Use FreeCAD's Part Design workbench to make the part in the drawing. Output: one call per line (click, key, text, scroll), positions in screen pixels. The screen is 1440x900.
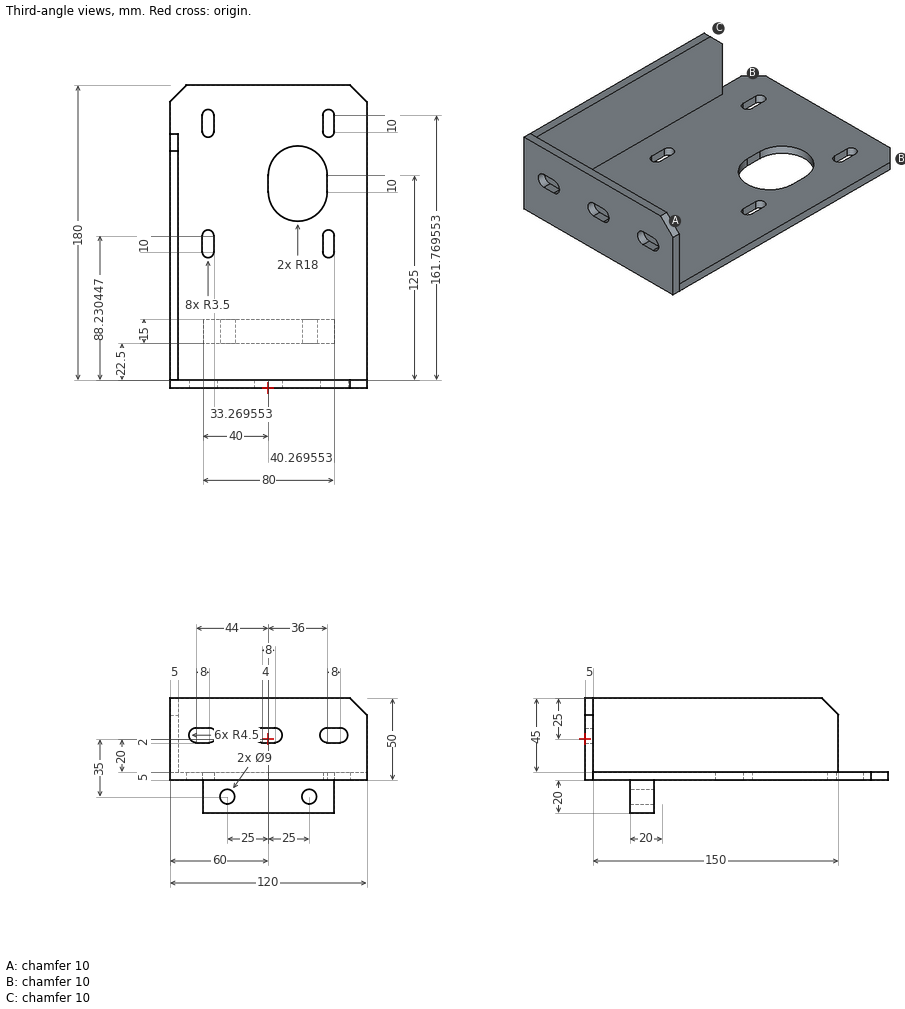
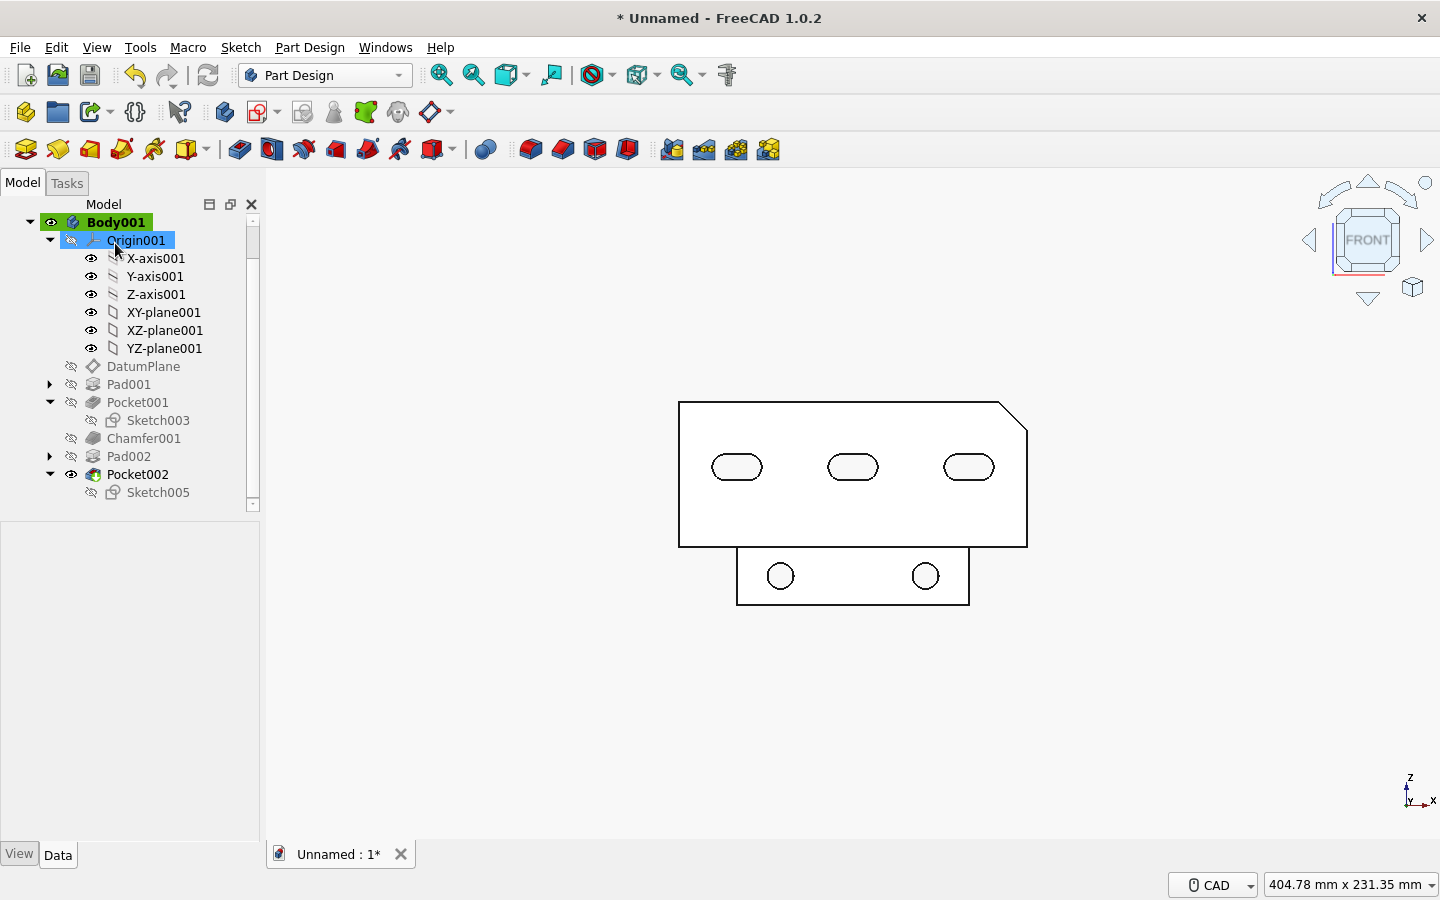
click(226, 112)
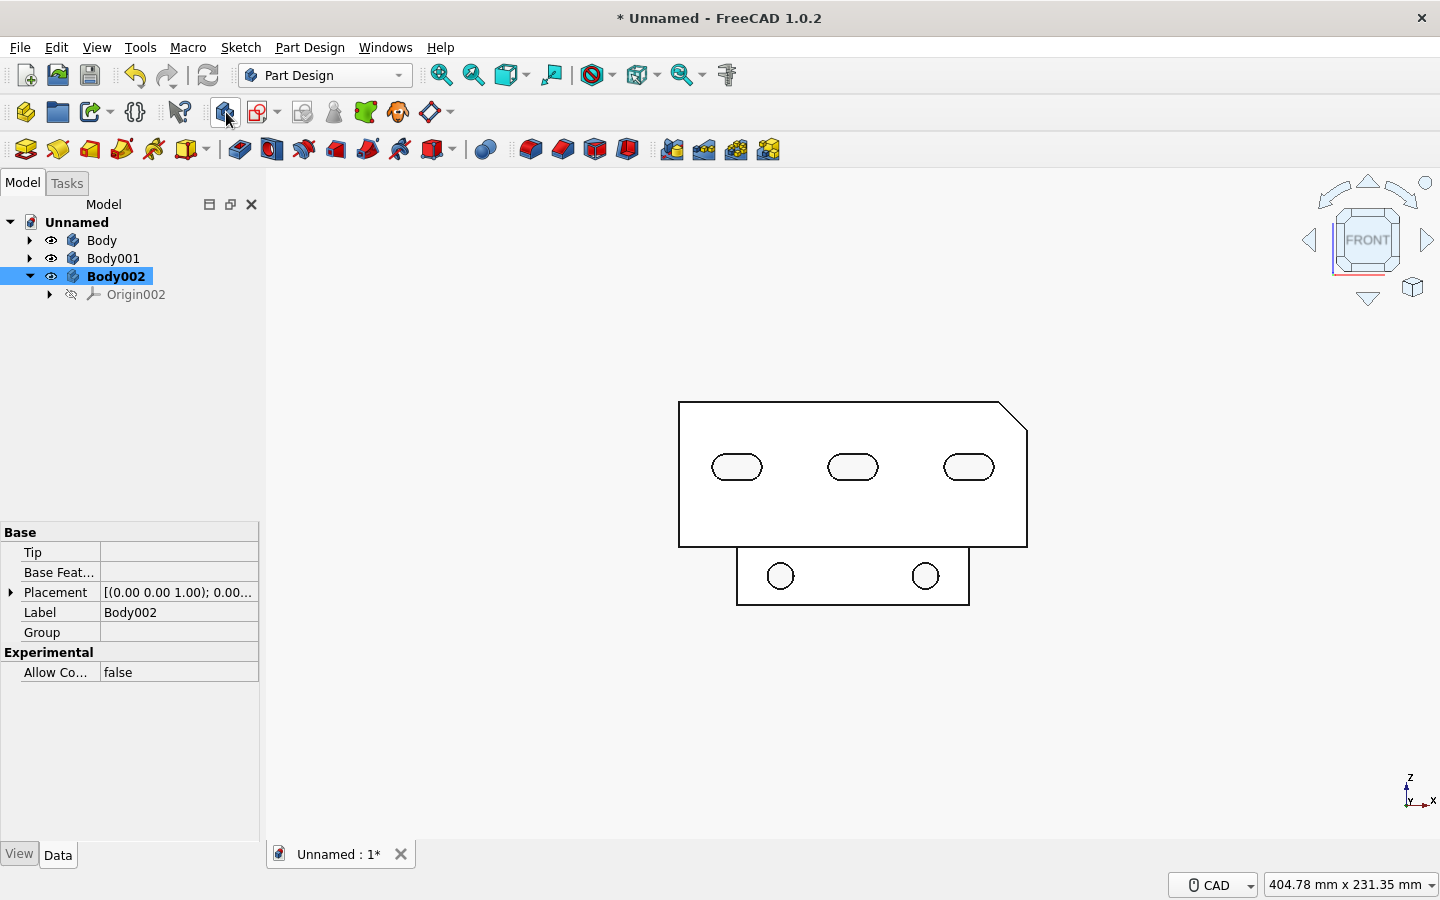
click(50, 294)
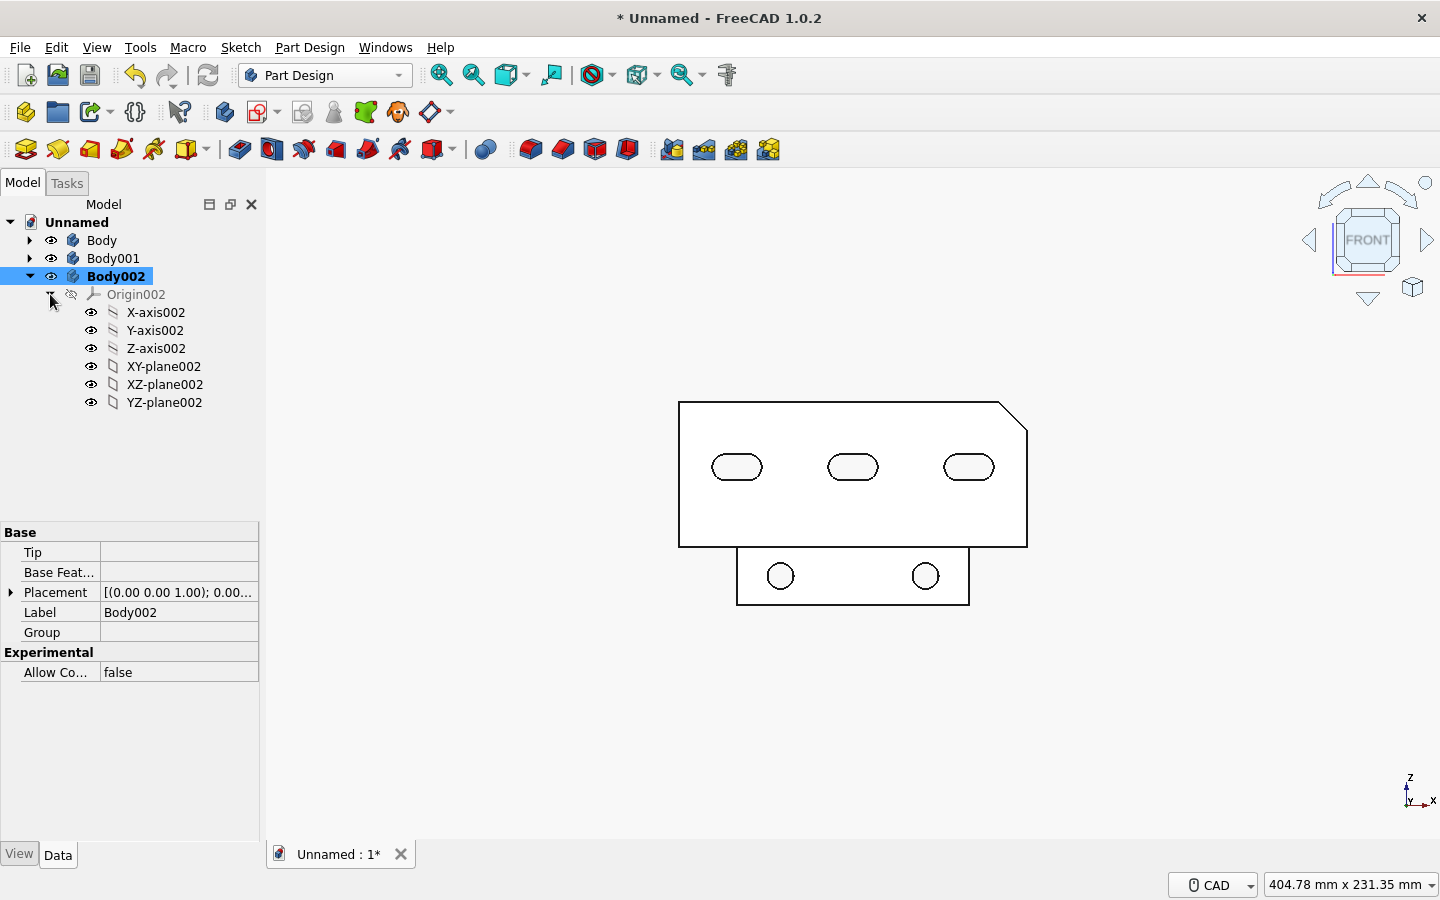
click(136, 402)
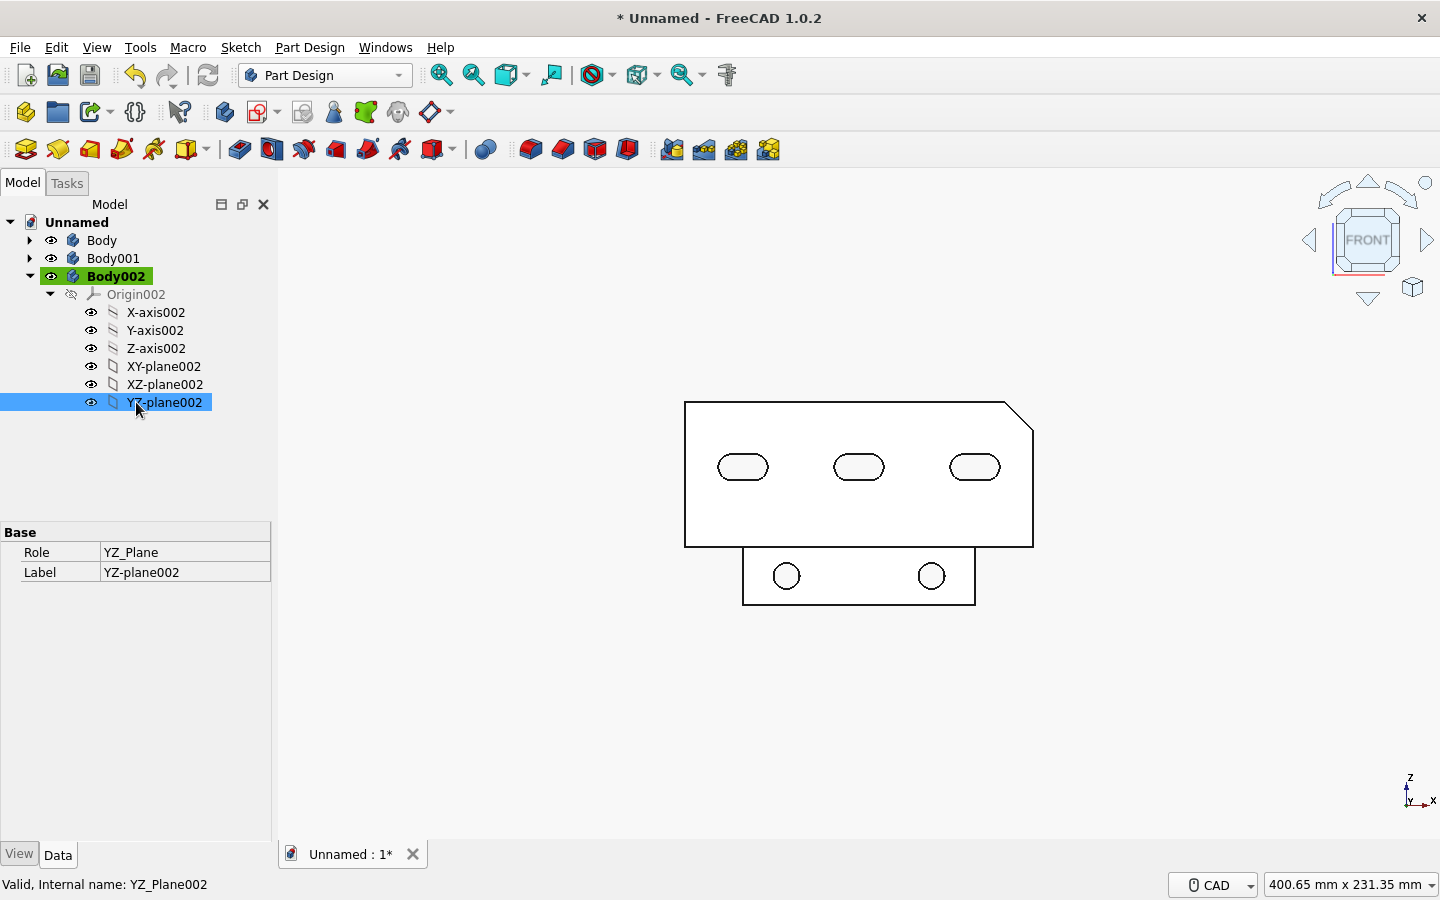
click(430, 112)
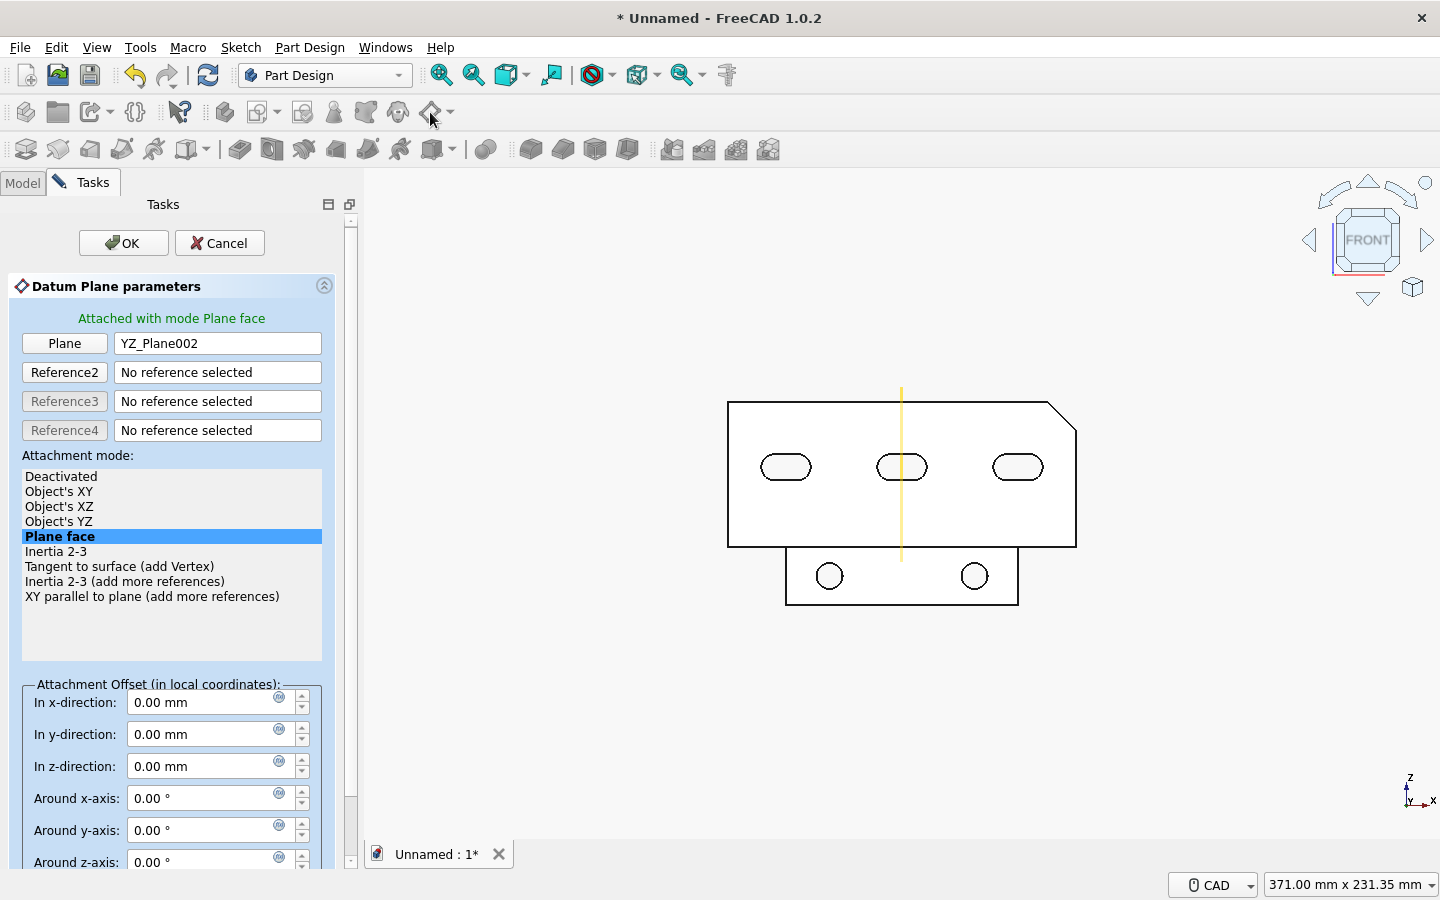
triple_click(210, 766)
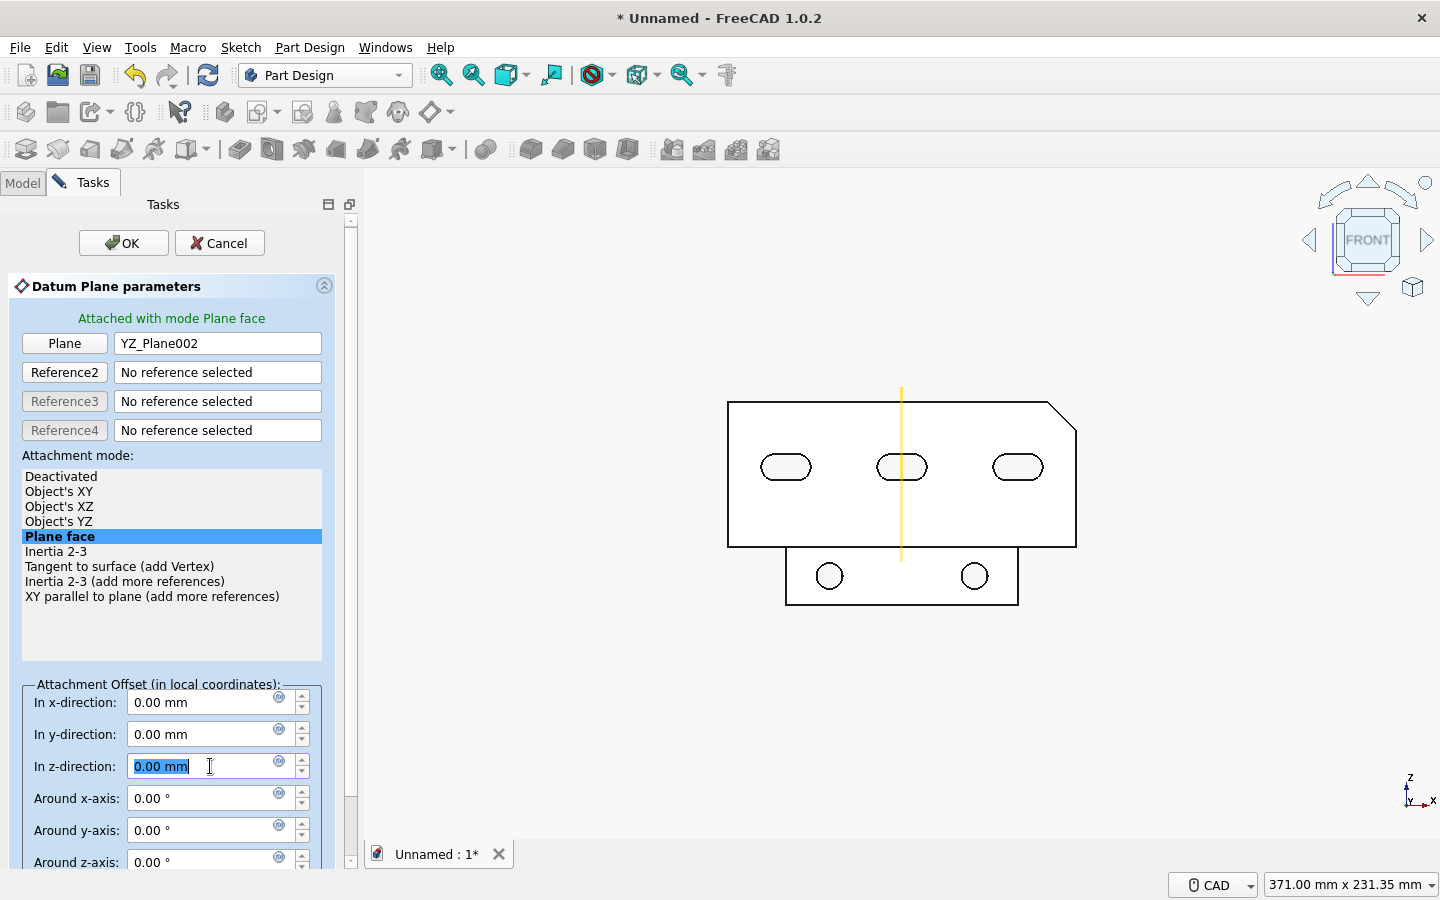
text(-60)
key(Tab)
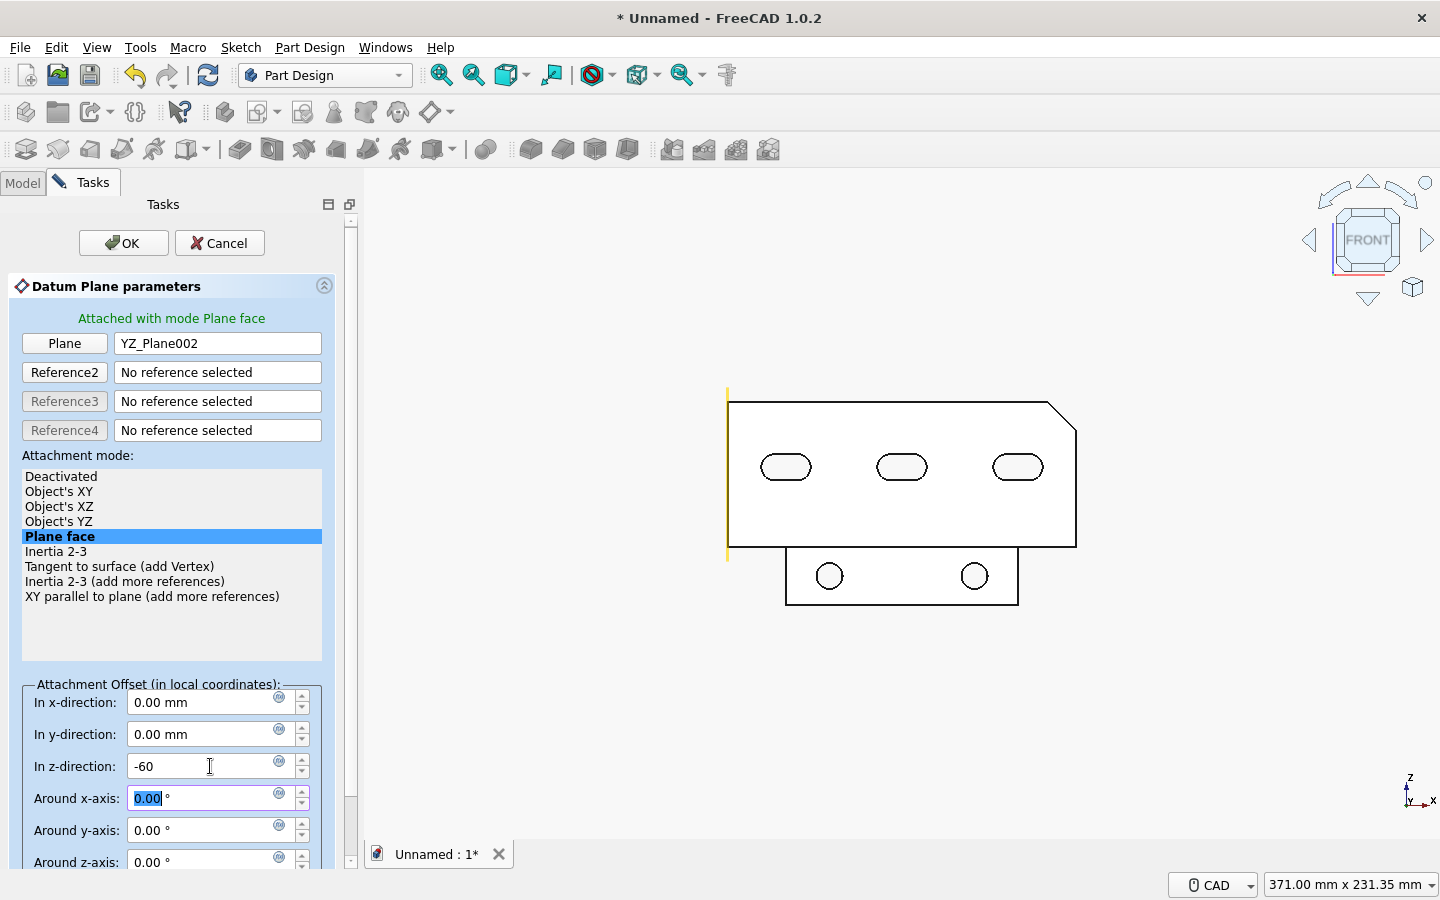
click(124, 243)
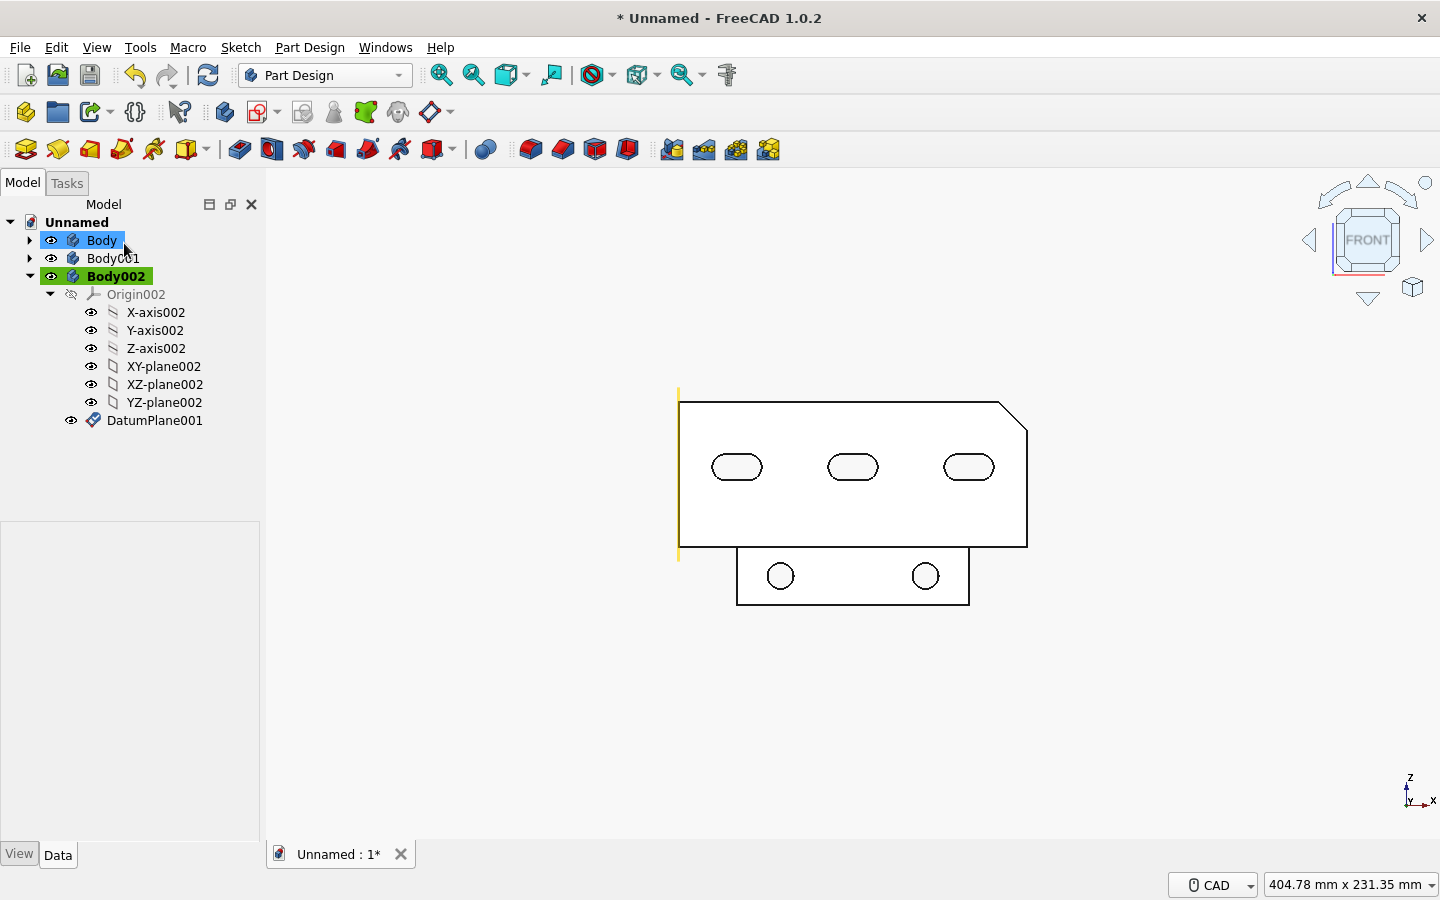
click(116, 420)